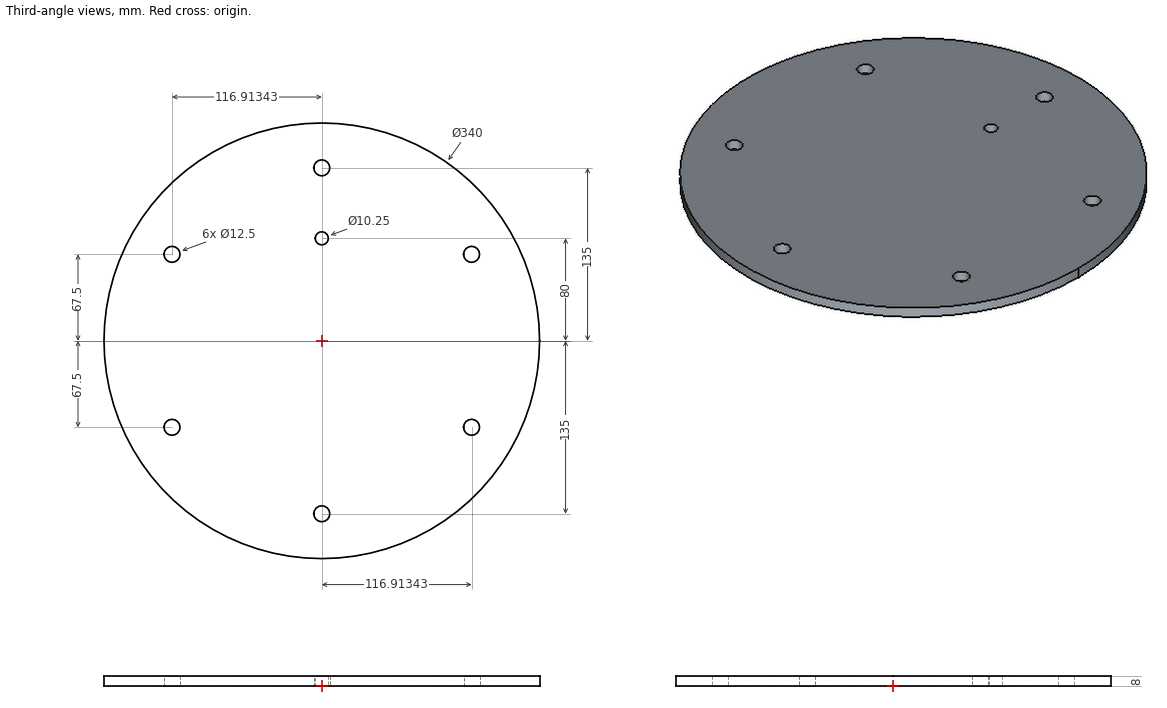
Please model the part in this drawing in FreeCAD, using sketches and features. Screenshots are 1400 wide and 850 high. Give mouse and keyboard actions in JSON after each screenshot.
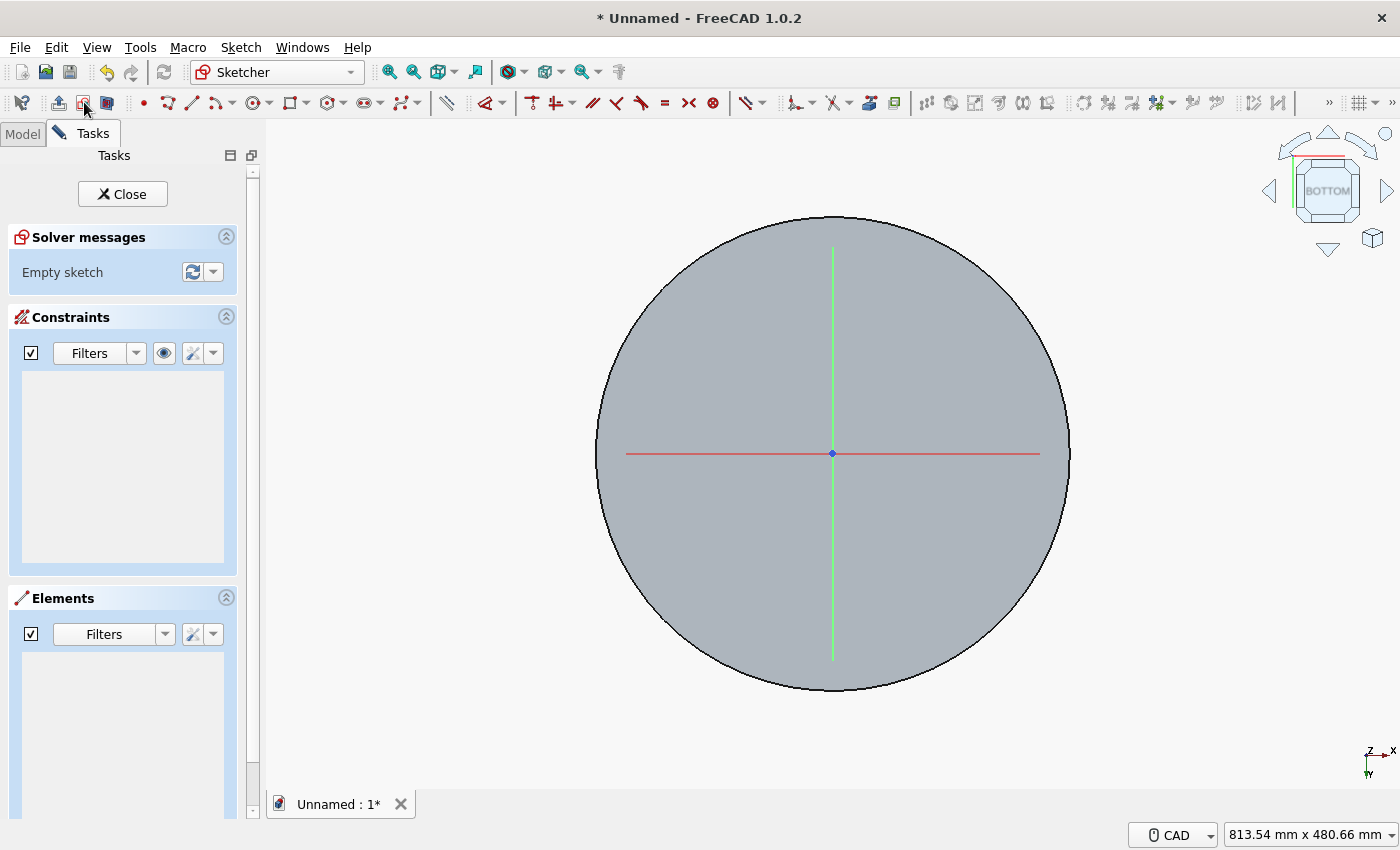
{"action": "left_click", "coordinate": [254, 104]}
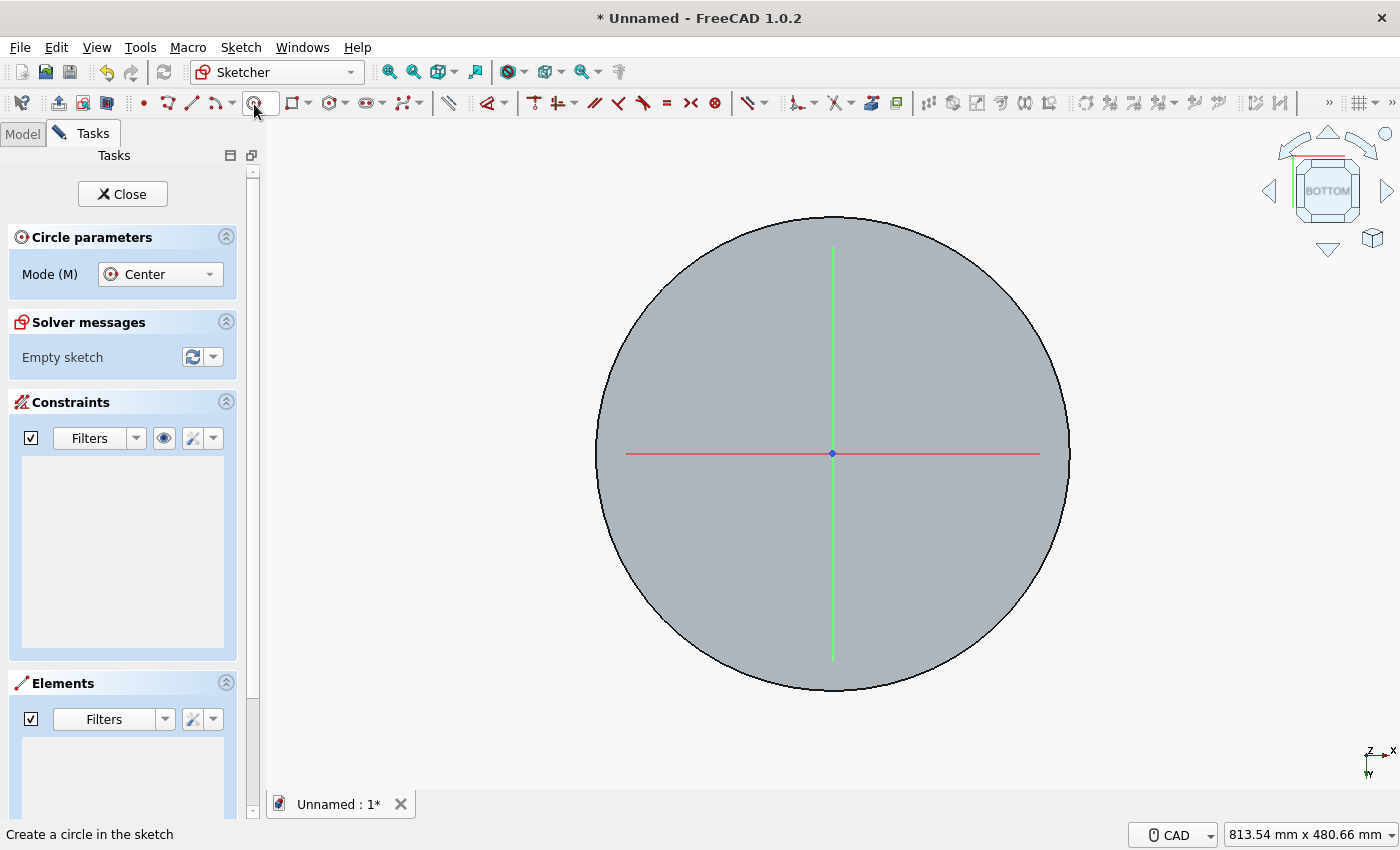
{"action": "scroll", "coordinate": [670, 548], "scroll_direction": "up", "scroll_amount": 5}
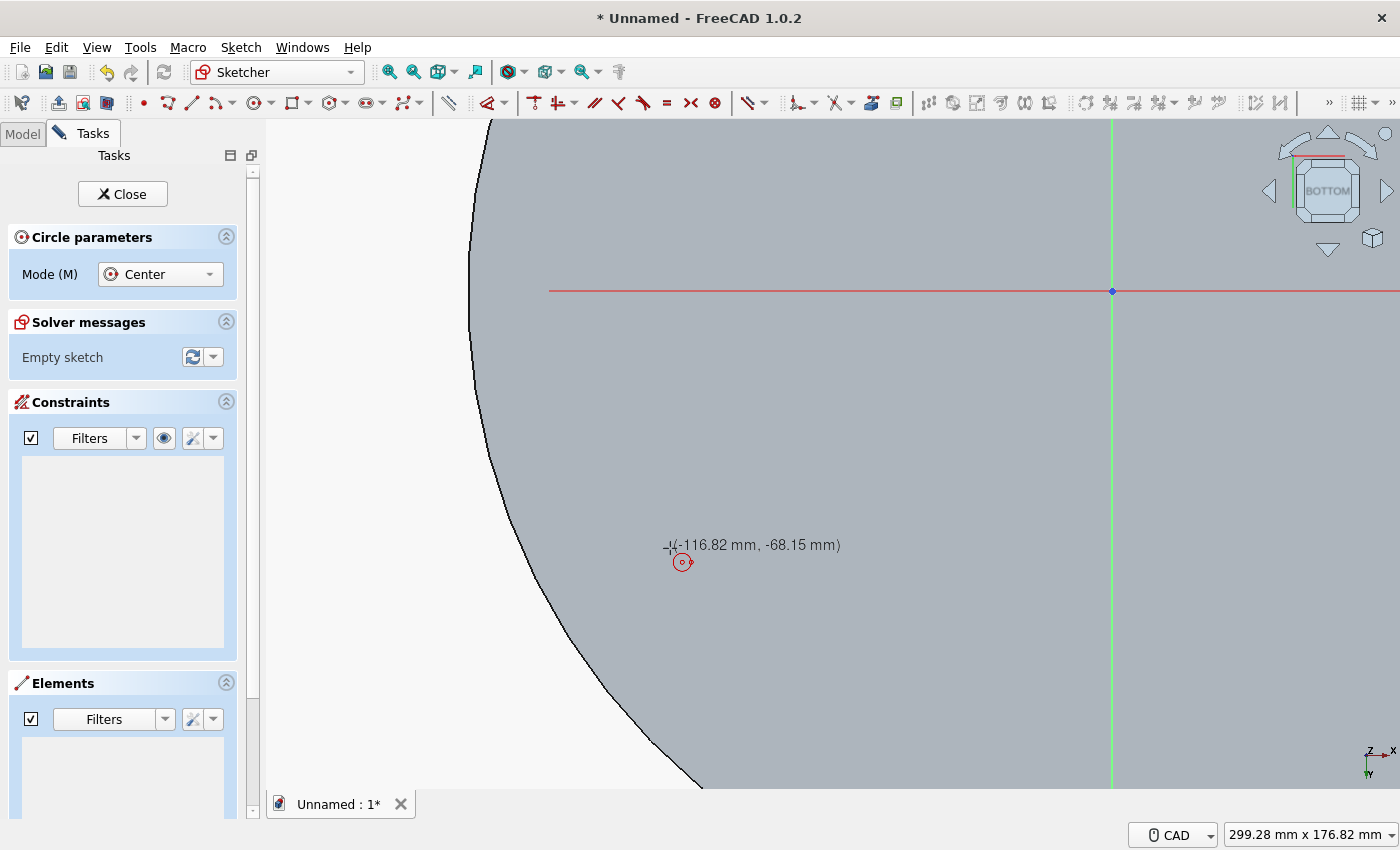
{"action": "left_click", "coordinate": [669, 547]}
{"action": "mouse_move", "coordinate": [686, 530]}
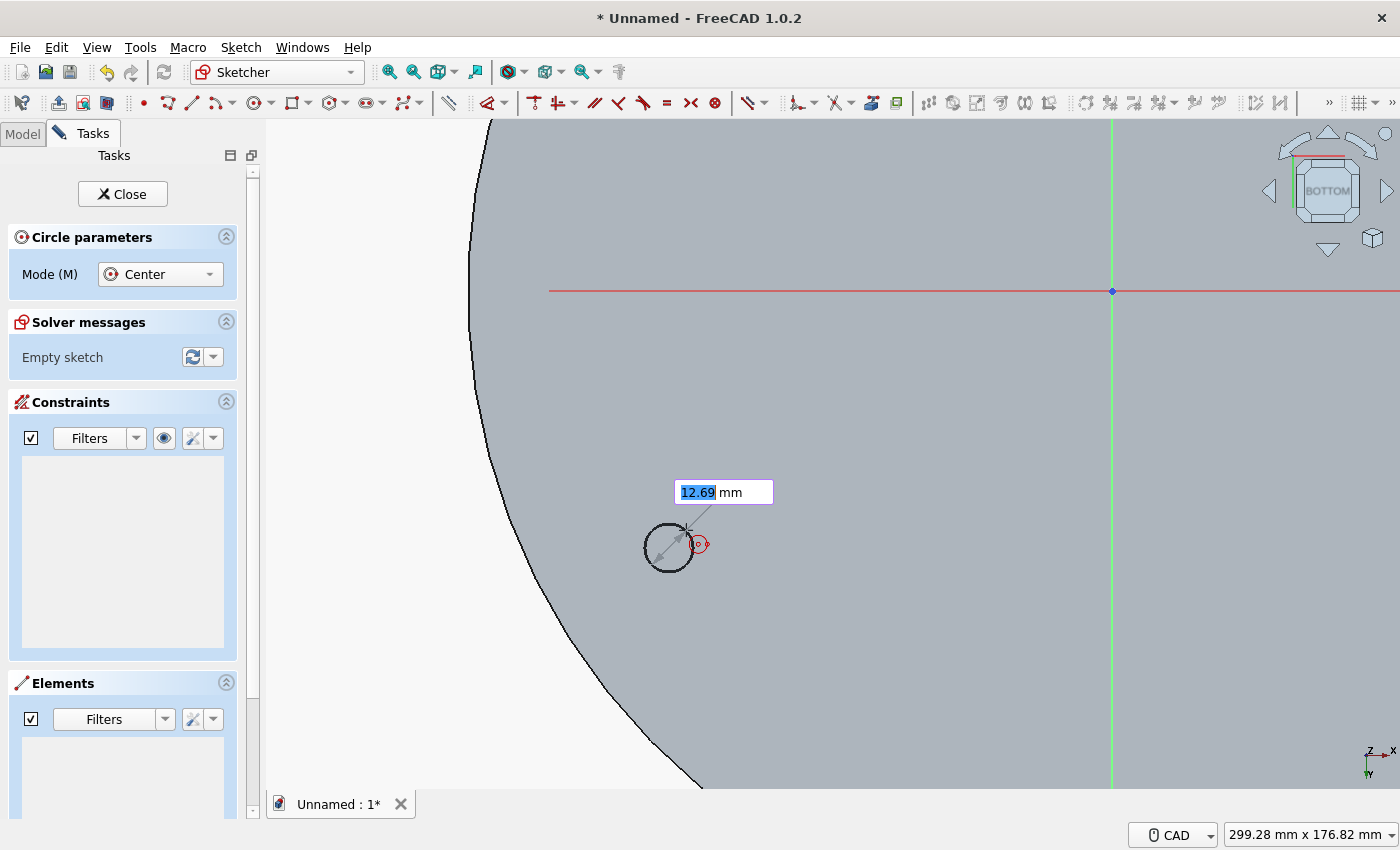
{"action": "type", "text": "12.5"}
{"action": "key", "text": "Return"}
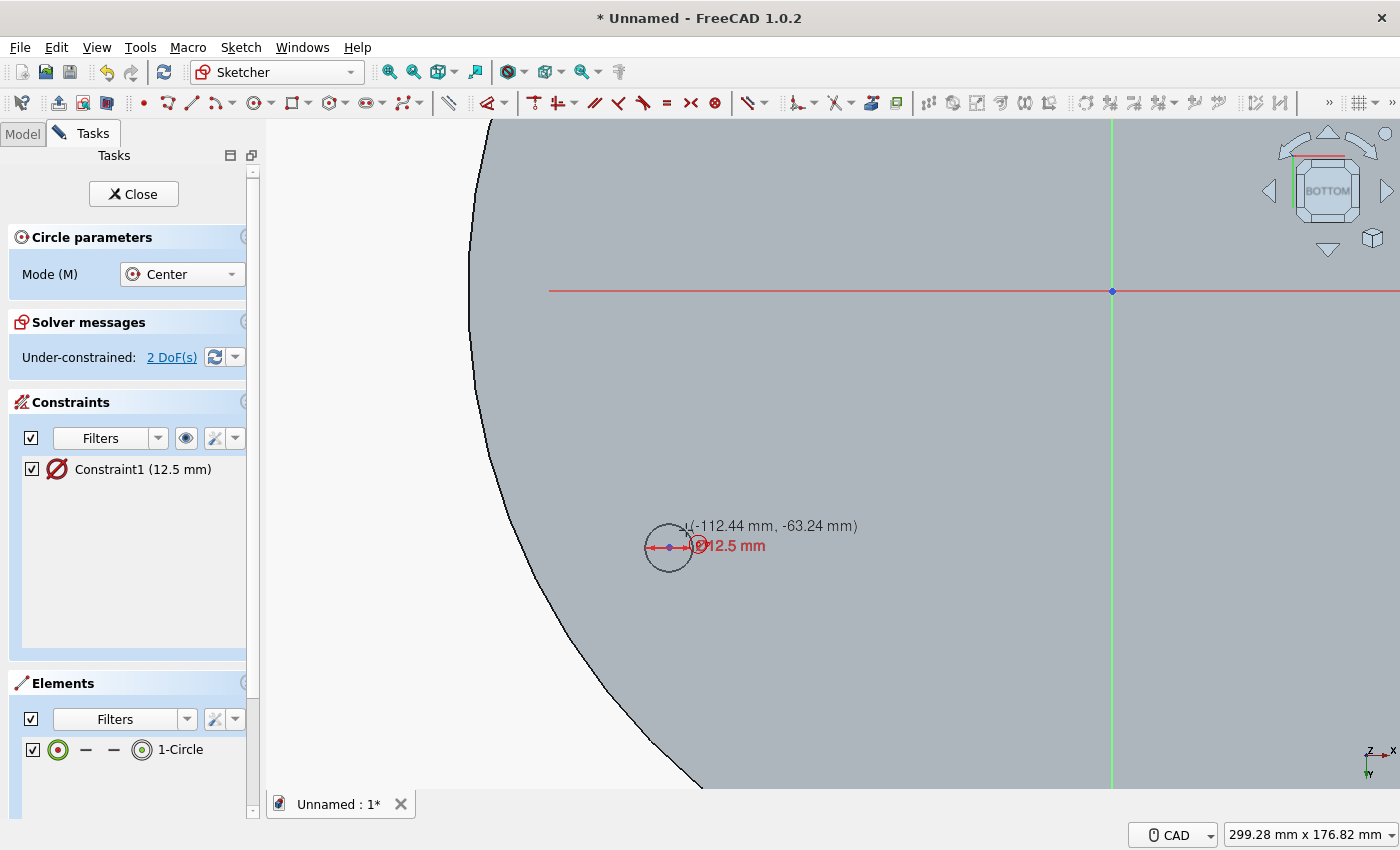
{"action": "scroll", "coordinate": [562, 549], "scroll_direction": "down", "scroll_amount": 5}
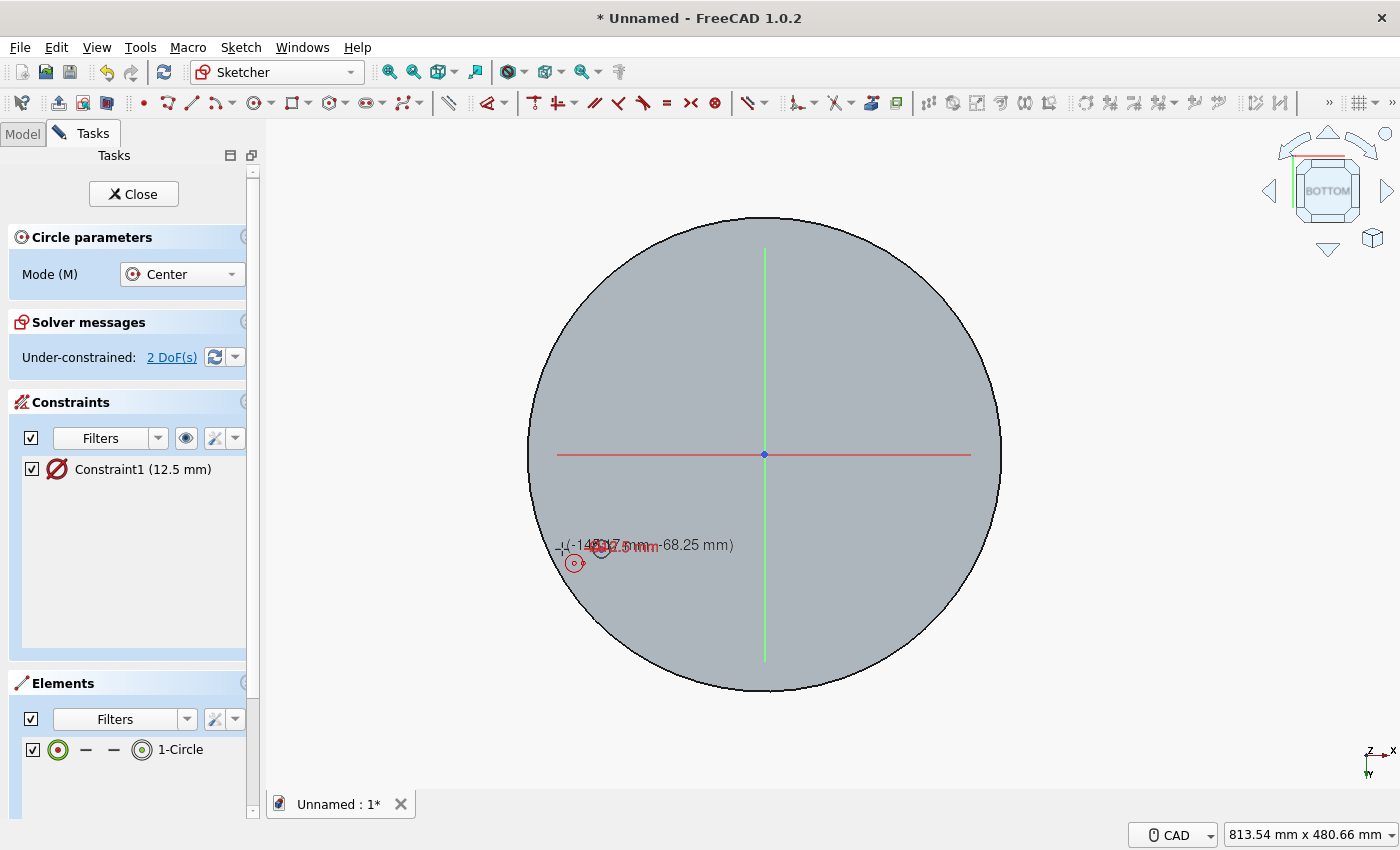
{"action": "scroll", "coordinate": [765, 643], "scroll_direction": "up", "scroll_amount": 5}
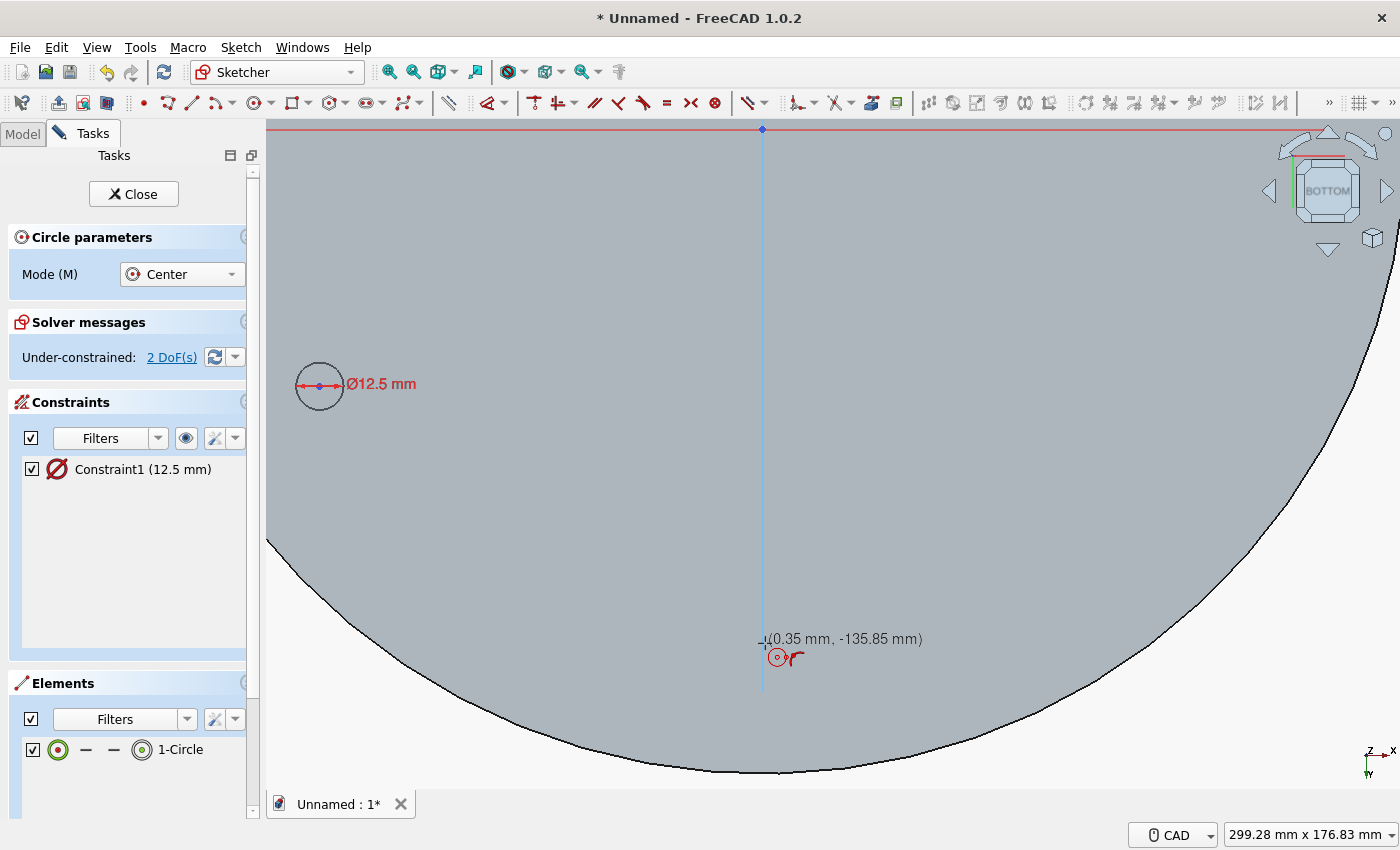
{"action": "left_click", "coordinate": [763, 641]}
{"action": "mouse_move", "coordinate": [780, 624]}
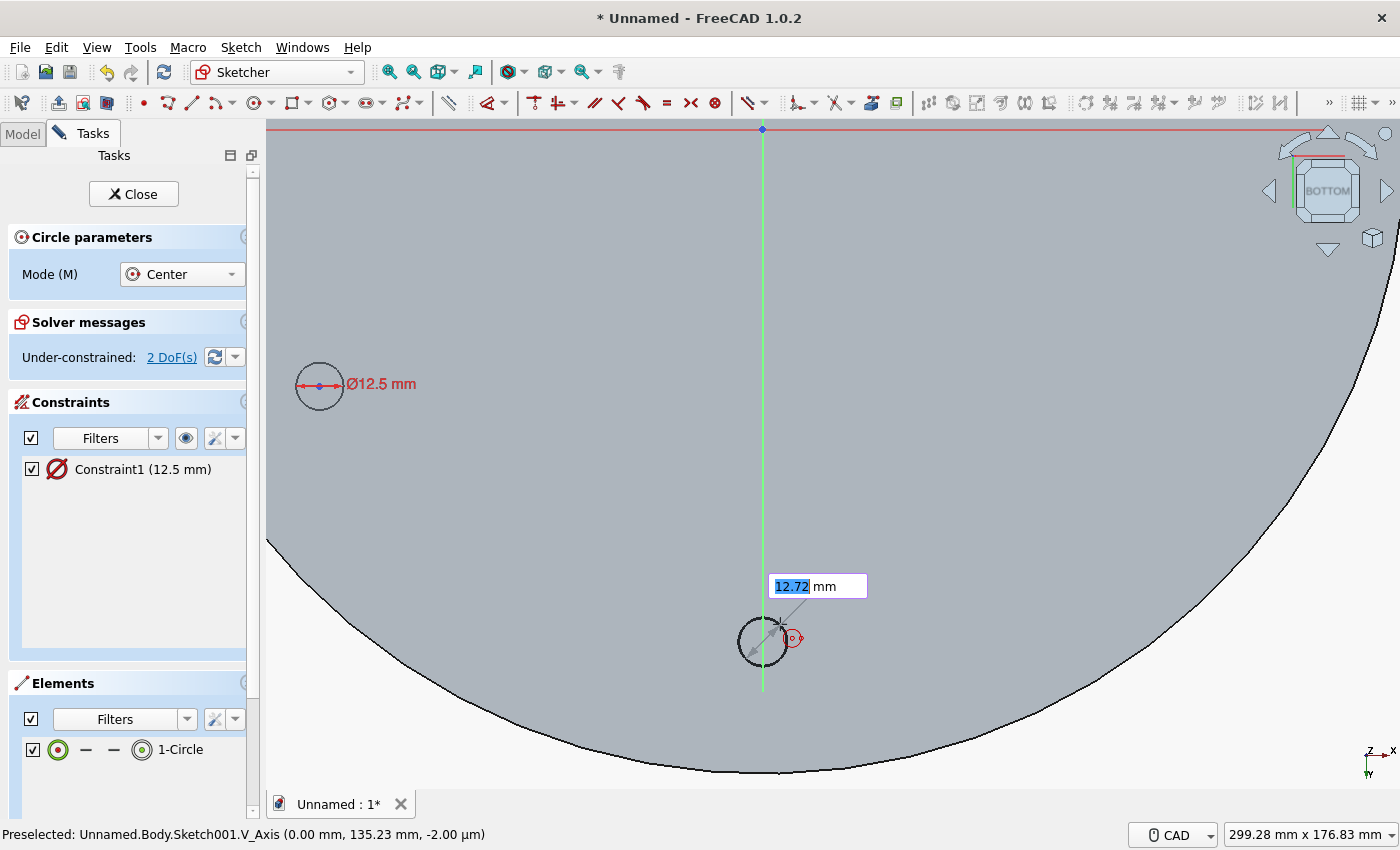
{"action": "type", "text": "12.5"}
{"action": "key", "text": "Return"}